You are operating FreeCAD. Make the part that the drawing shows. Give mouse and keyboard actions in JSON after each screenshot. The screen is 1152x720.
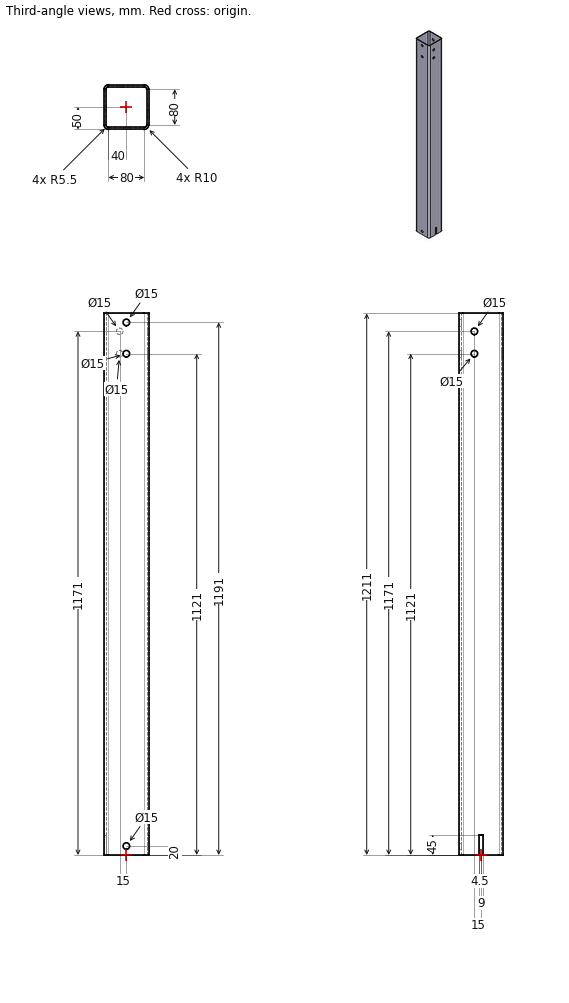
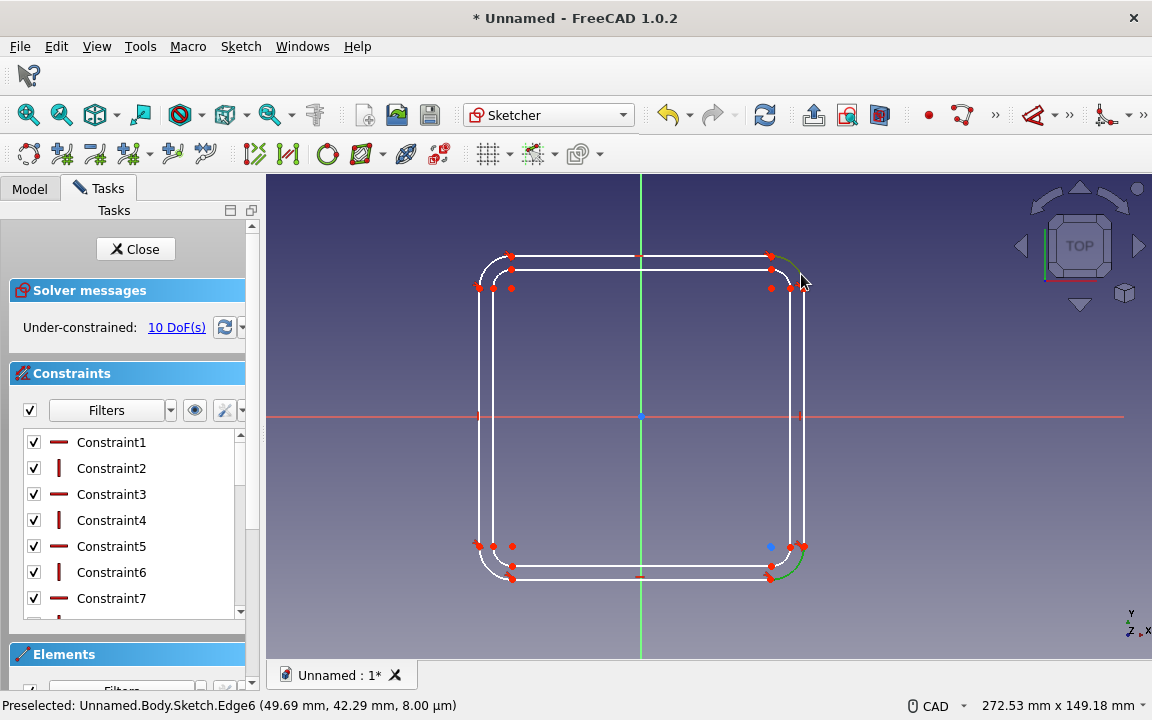
{"action": "left_click", "coordinate": [497, 260]}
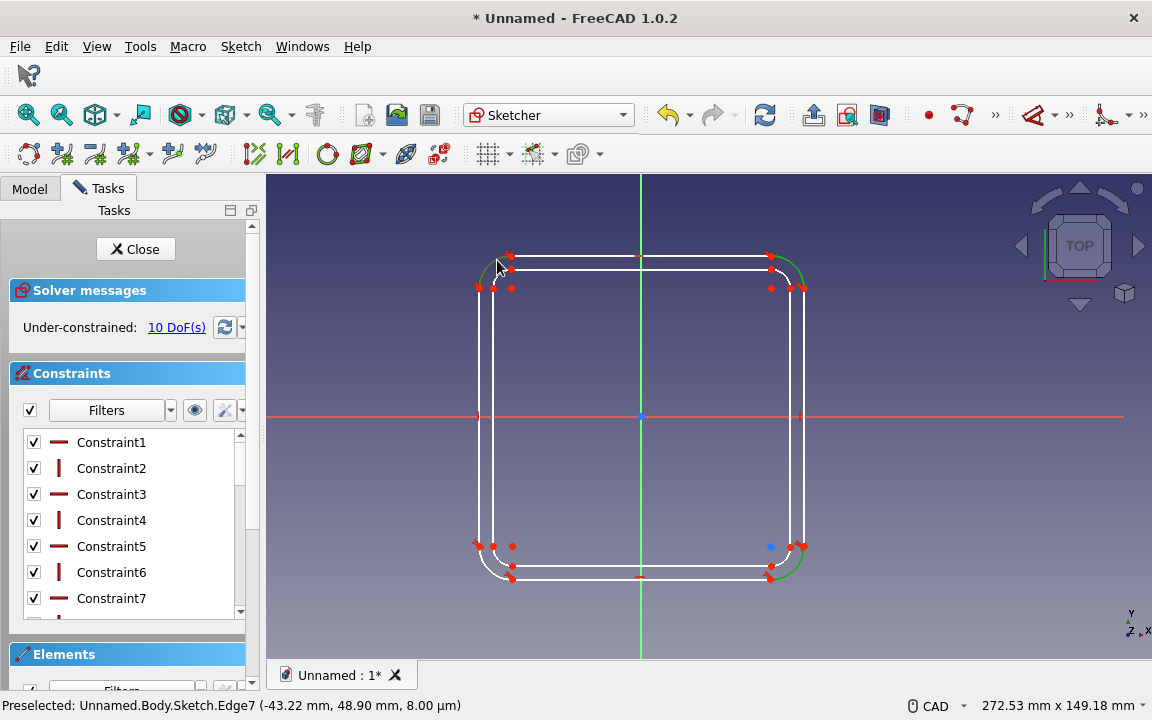
{"action": "left_click", "coordinate": [483, 562]}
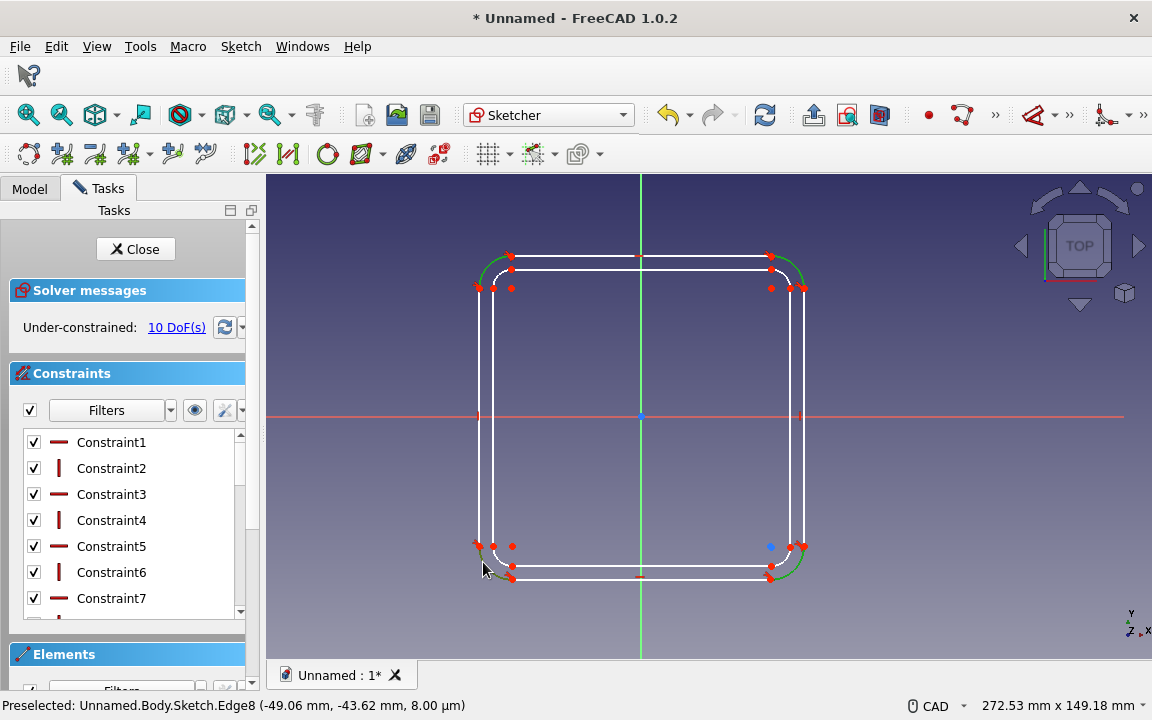
{"action": "key", "text": "e"}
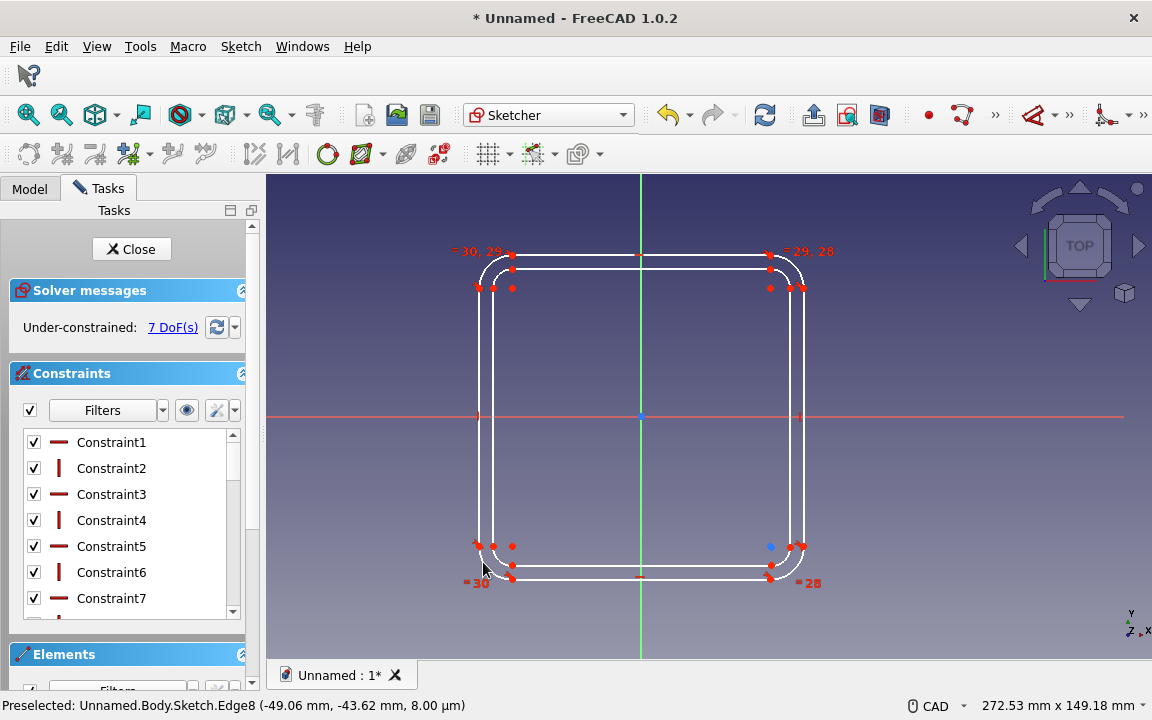
{"action": "scroll", "coordinate": [495, 555], "scroll_direction": "up", "scroll_amount": 3}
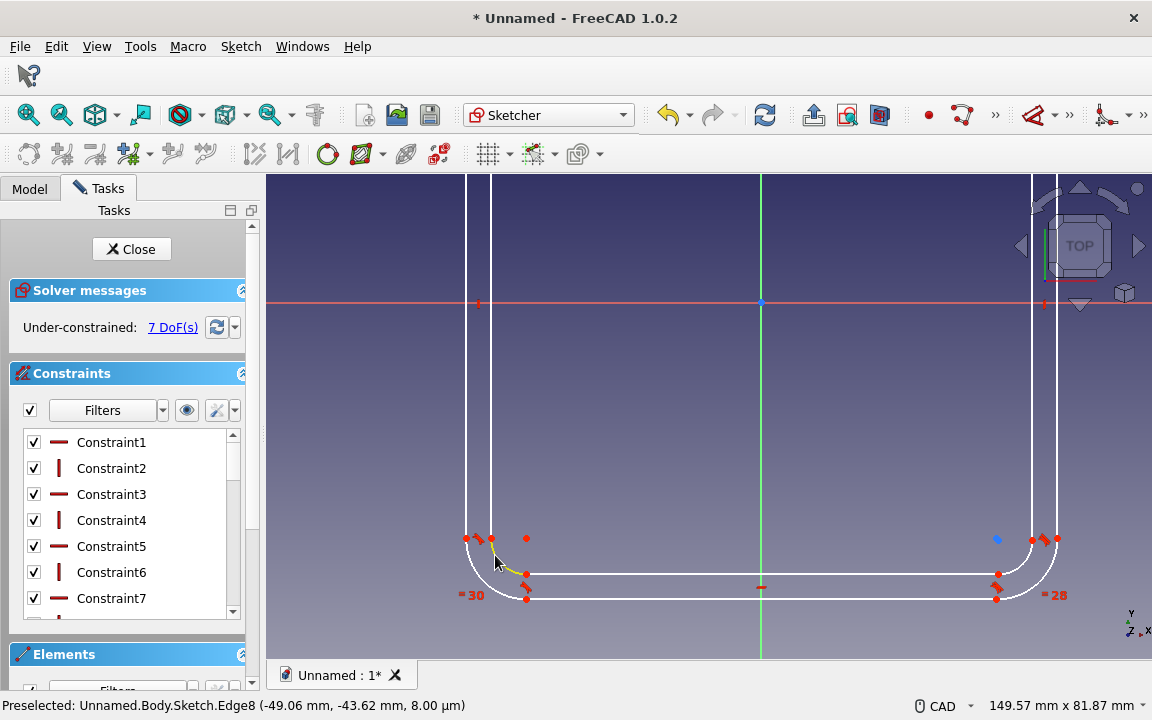
{"action": "left_click", "coordinate": [495, 555]}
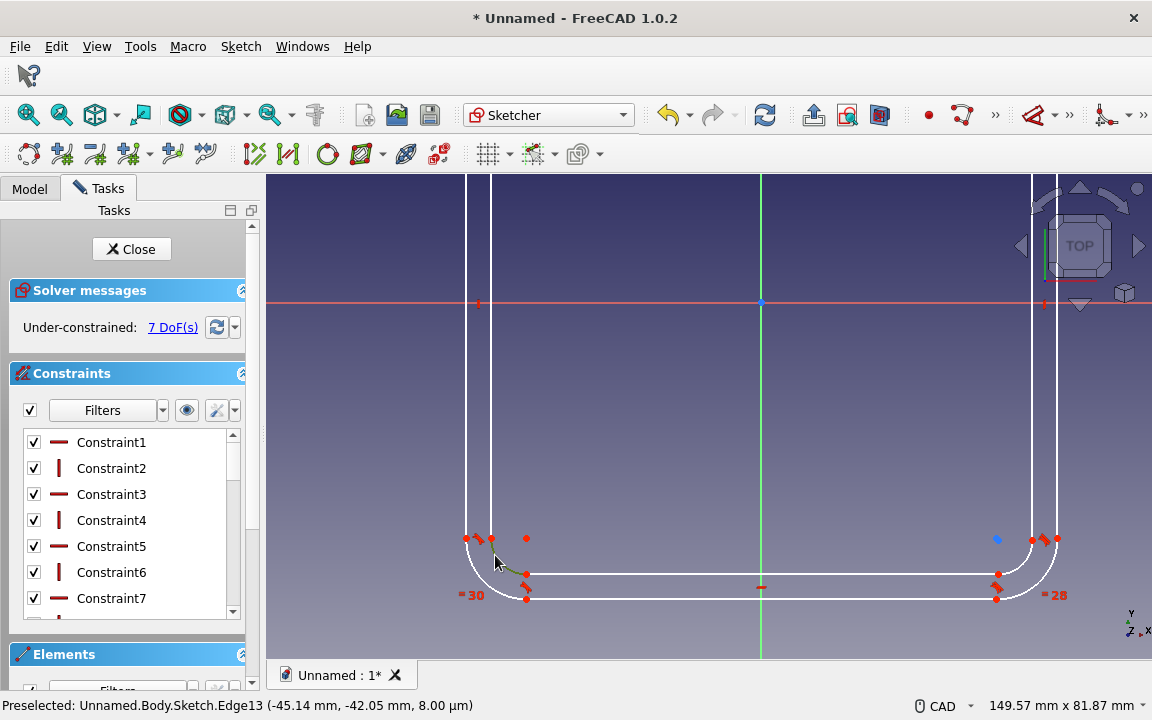
{"action": "scroll", "coordinate": [494, 555], "scroll_direction": "down", "scroll_amount": 3}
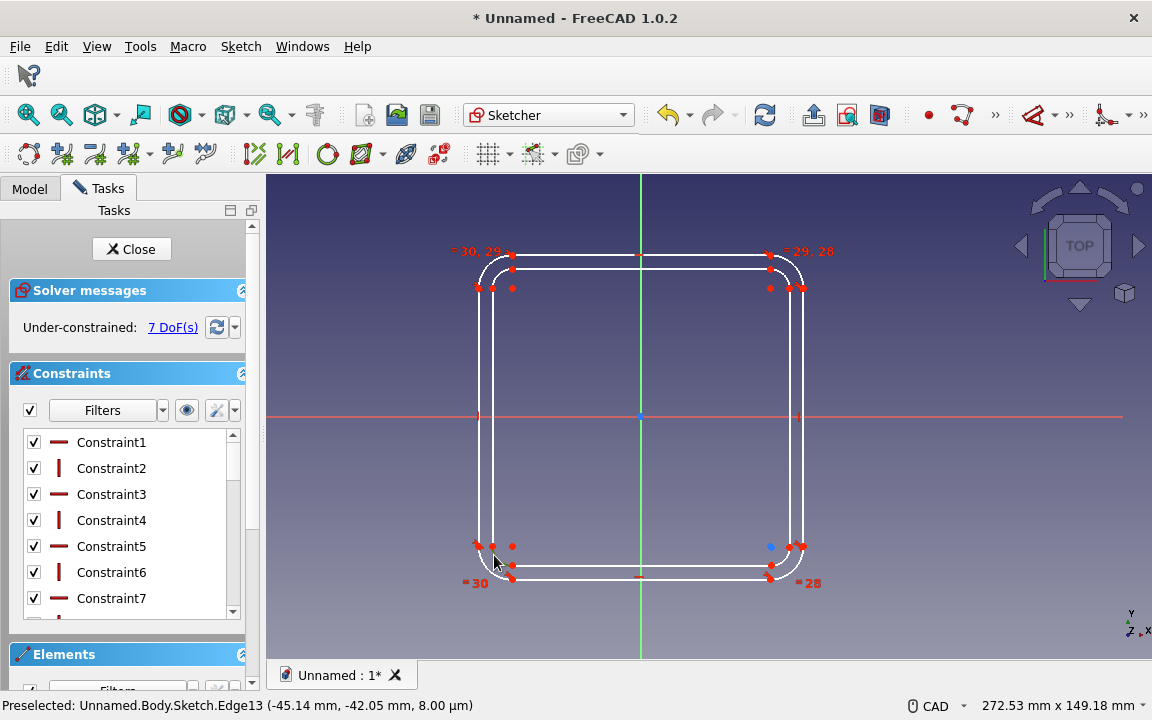
{"action": "scroll", "coordinate": [779, 564], "scroll_direction": "up", "scroll_amount": 3}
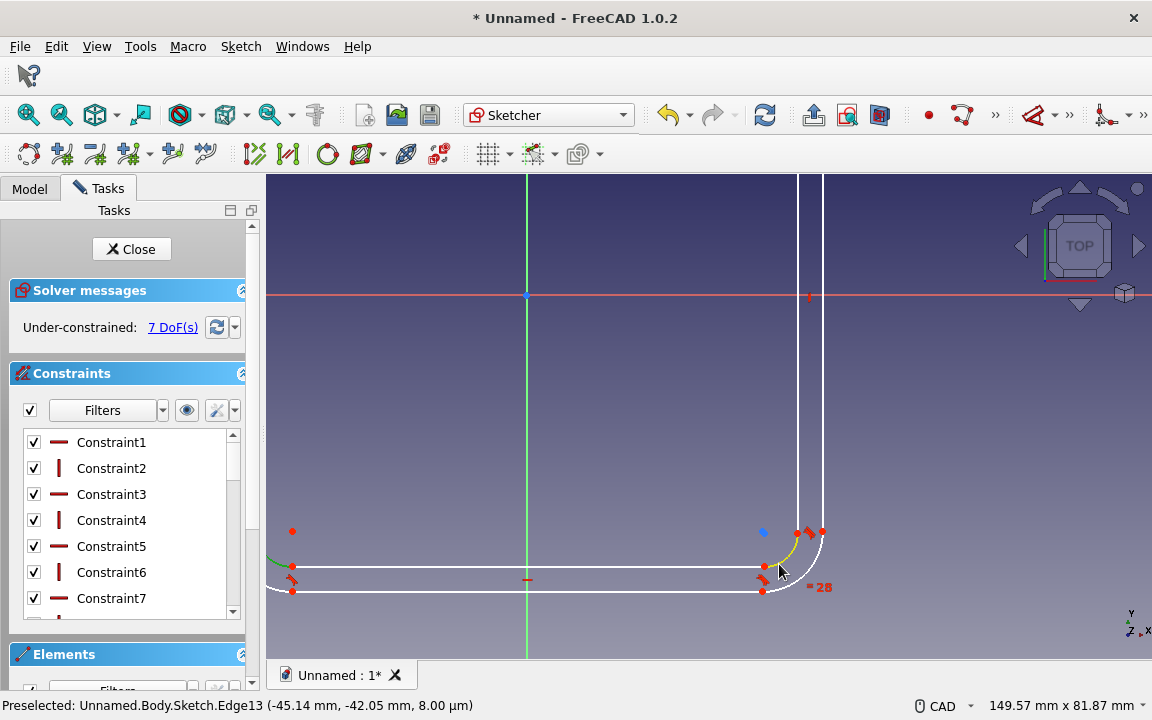
{"action": "left_click", "coordinate": [779, 563]}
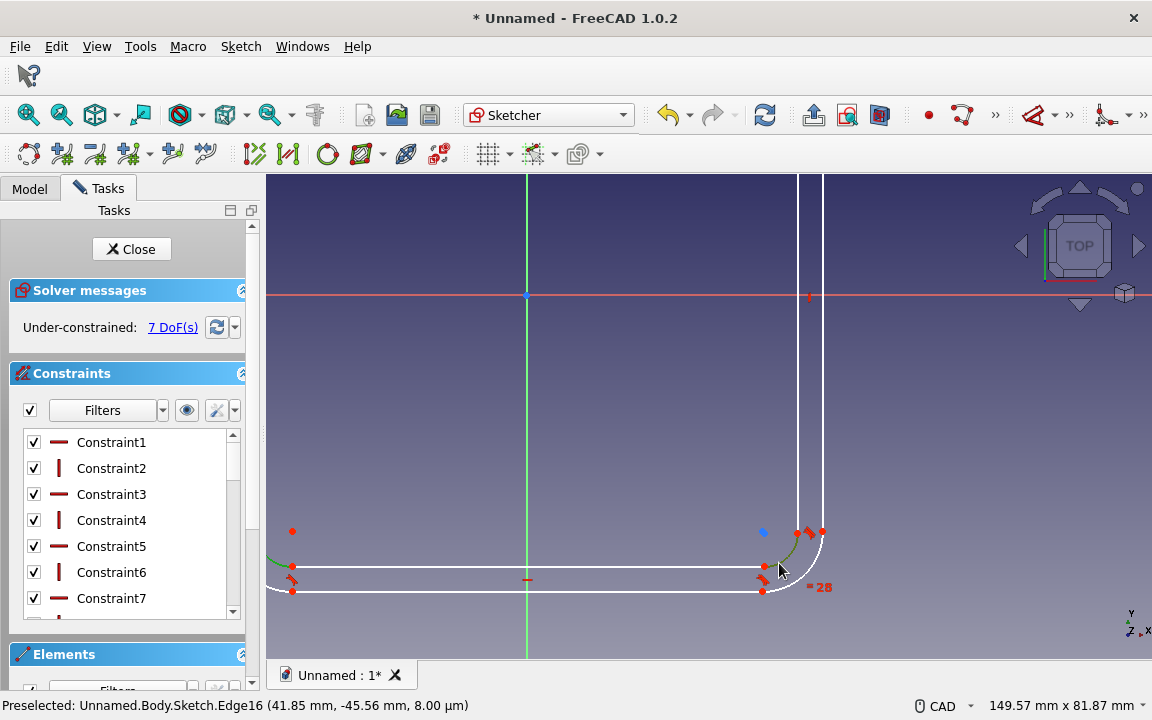
{"action": "key", "text": "e"}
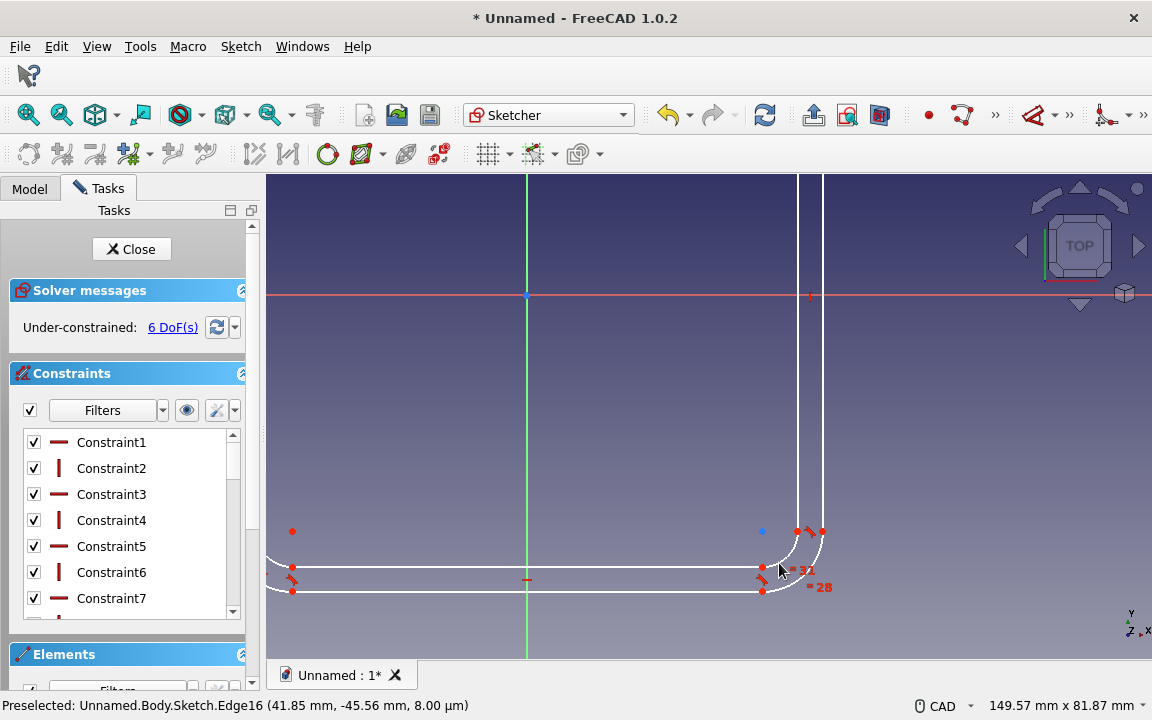
{"action": "key", "text": "d"}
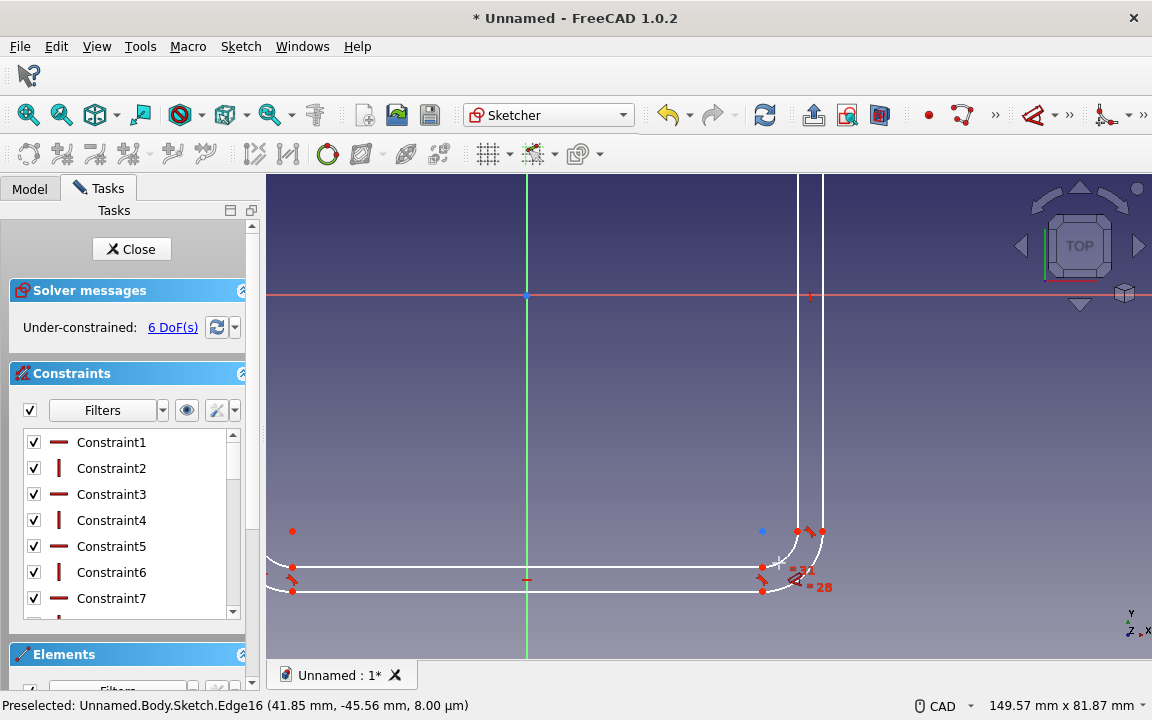
{"action": "left_click", "coordinate": [790, 585]}
{"action": "left_click", "coordinate": [805, 613]}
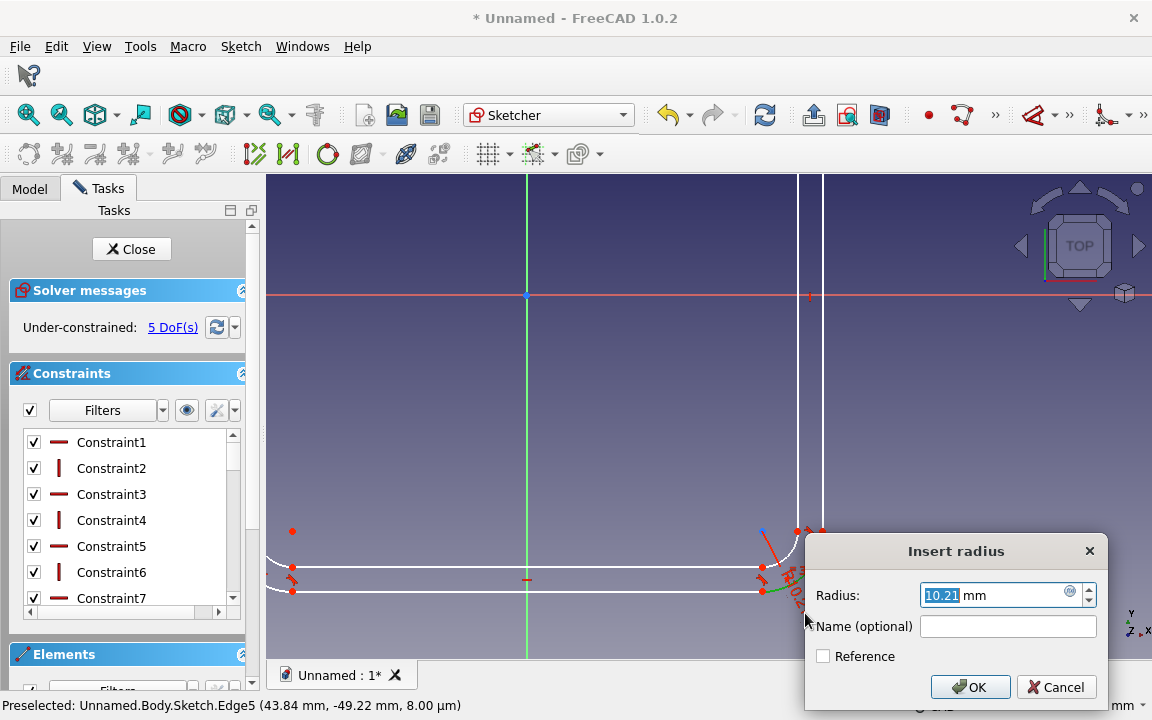
{"action": "type", "text": "10"}
{"action": "key", "text": "Return"}